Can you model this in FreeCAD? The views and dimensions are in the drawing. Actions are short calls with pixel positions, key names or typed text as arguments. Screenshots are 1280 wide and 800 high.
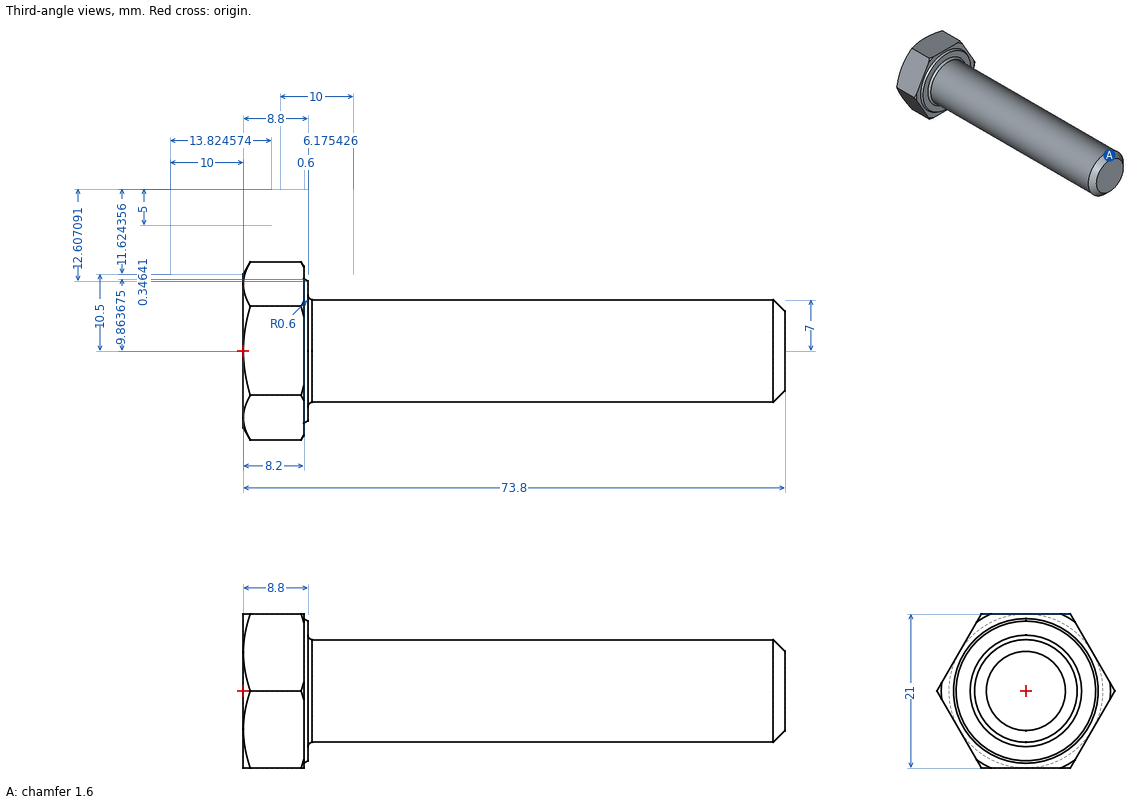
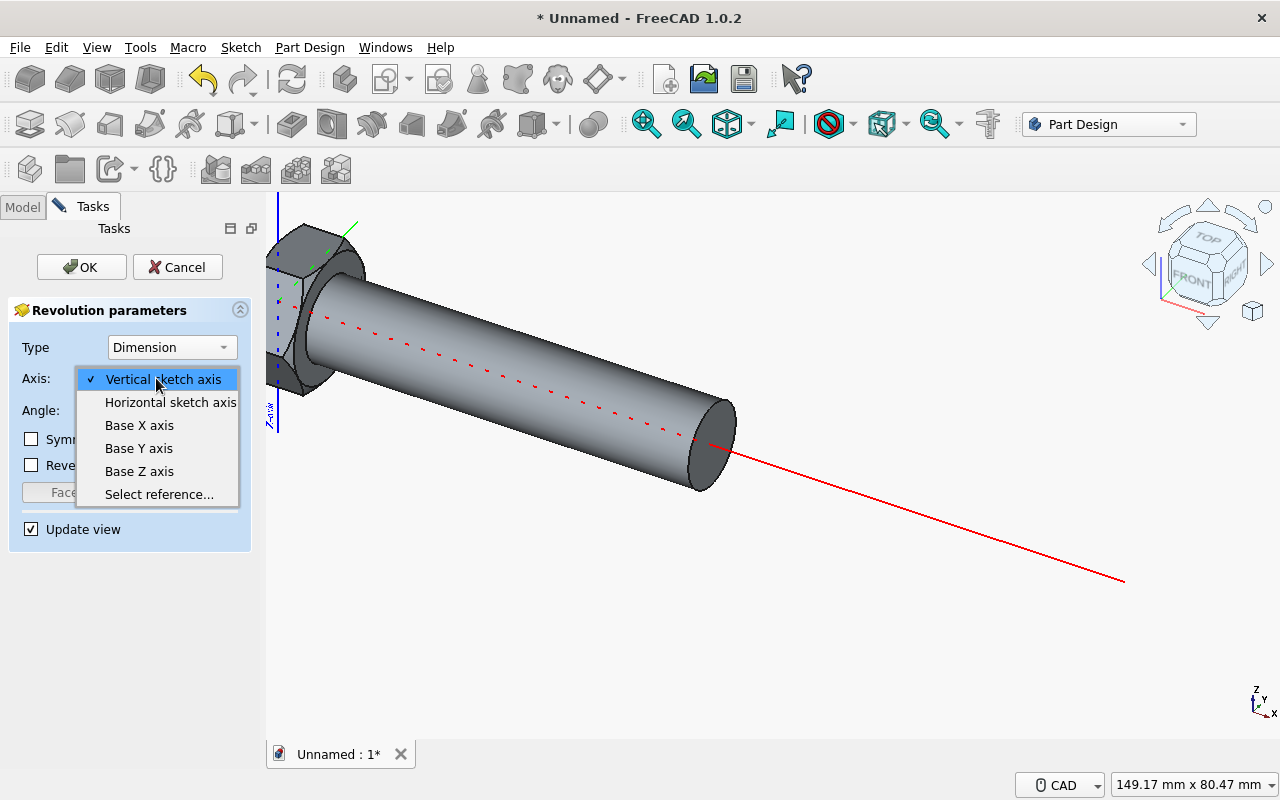
click(156, 402)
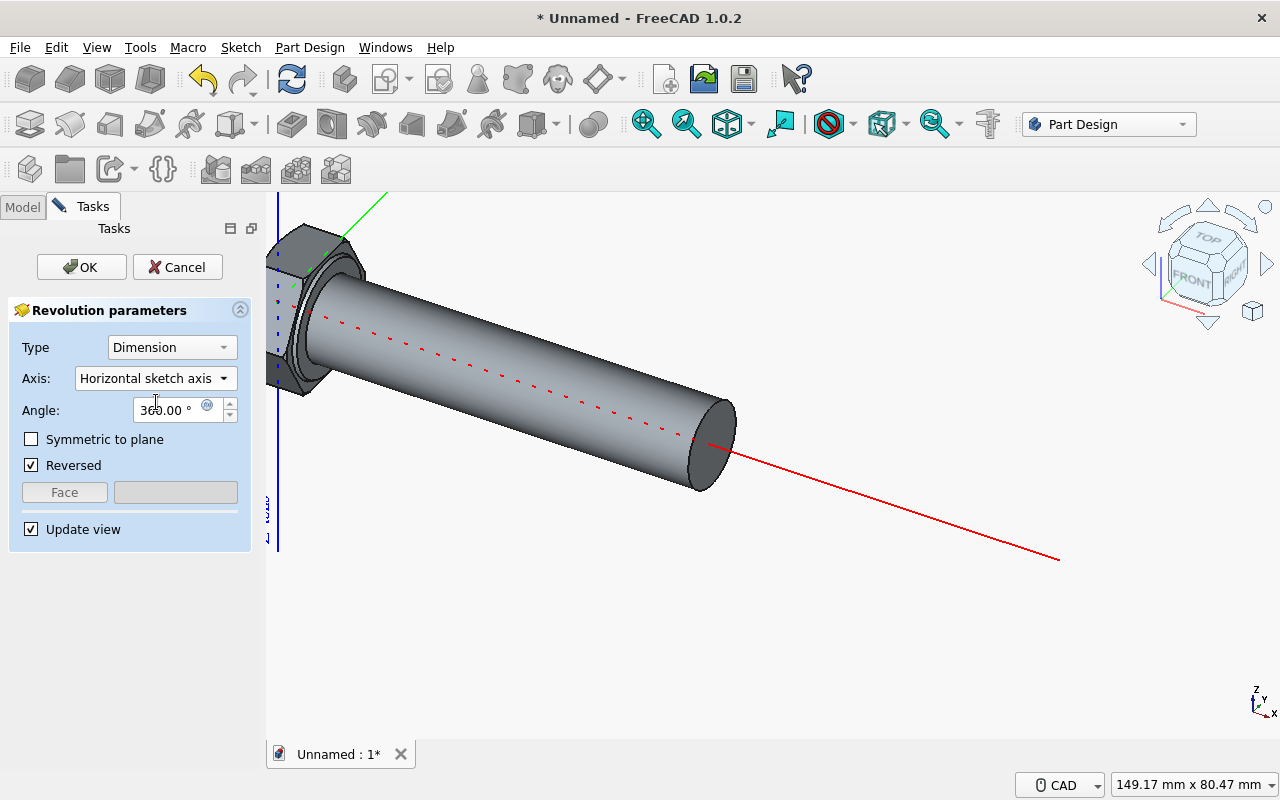
click(82, 267)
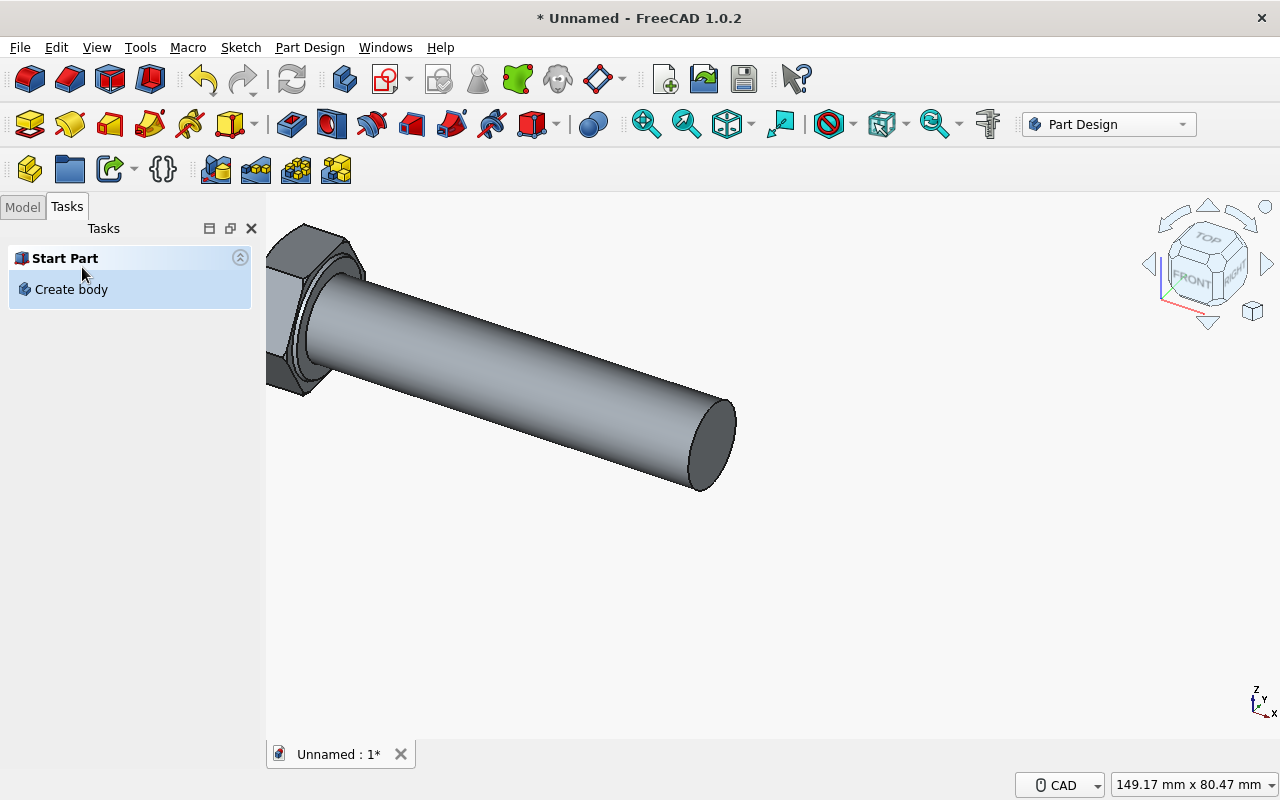
click(648, 124)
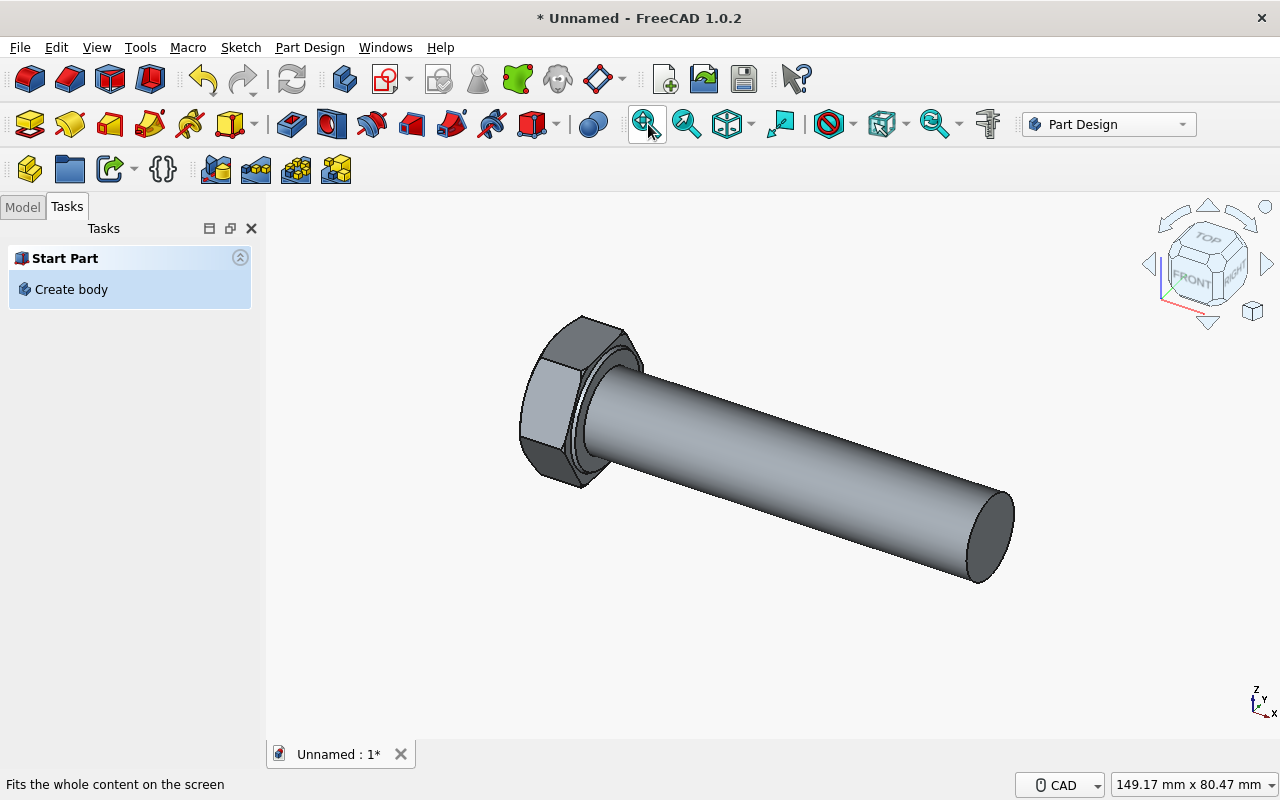
click(966, 560)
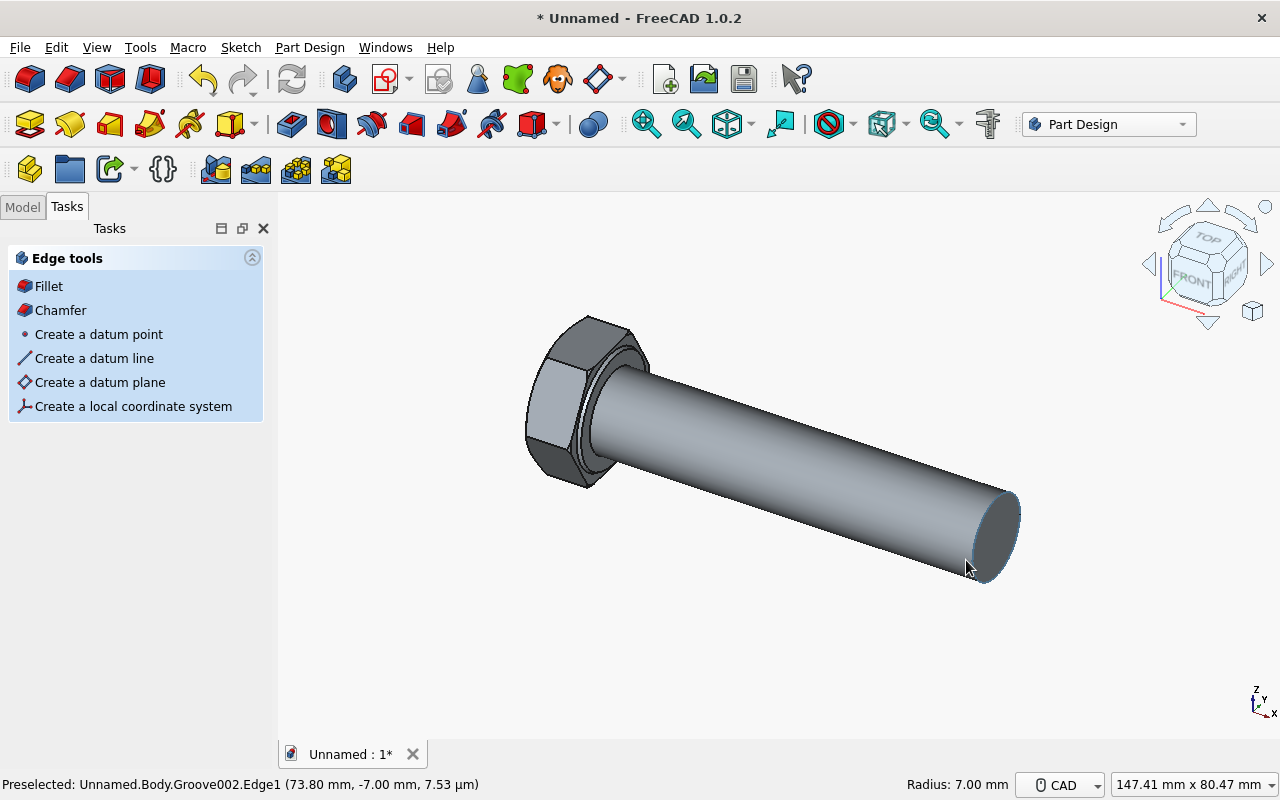
click(70, 80)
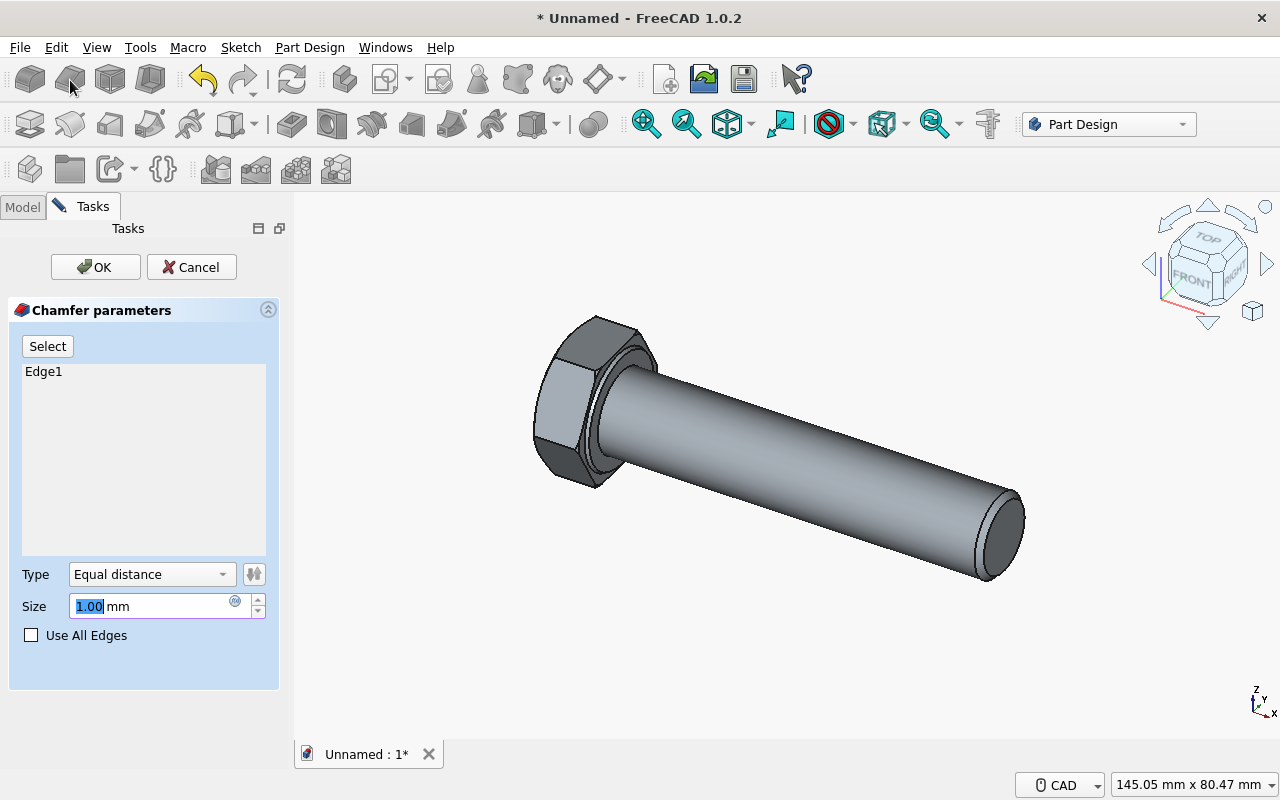
text(1.6)
key(Tab)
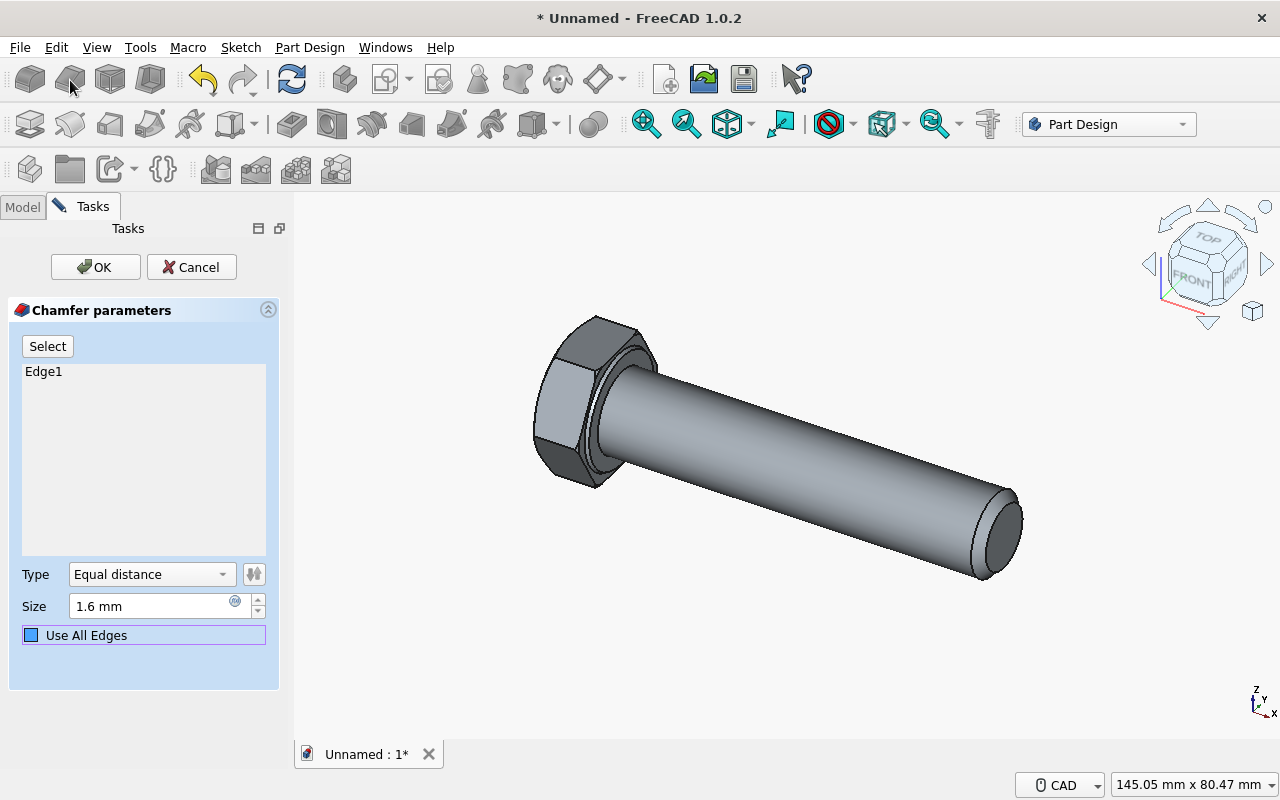
click(96, 267)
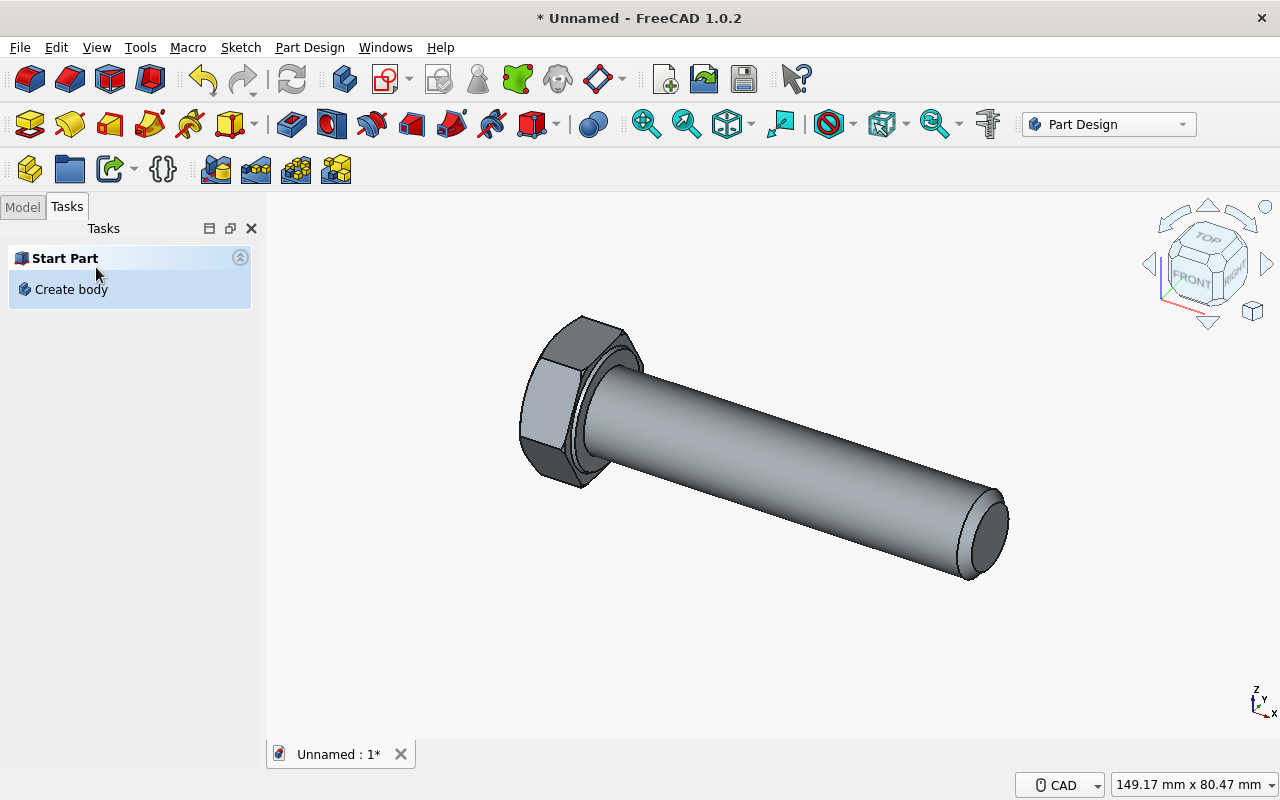
click(386, 80)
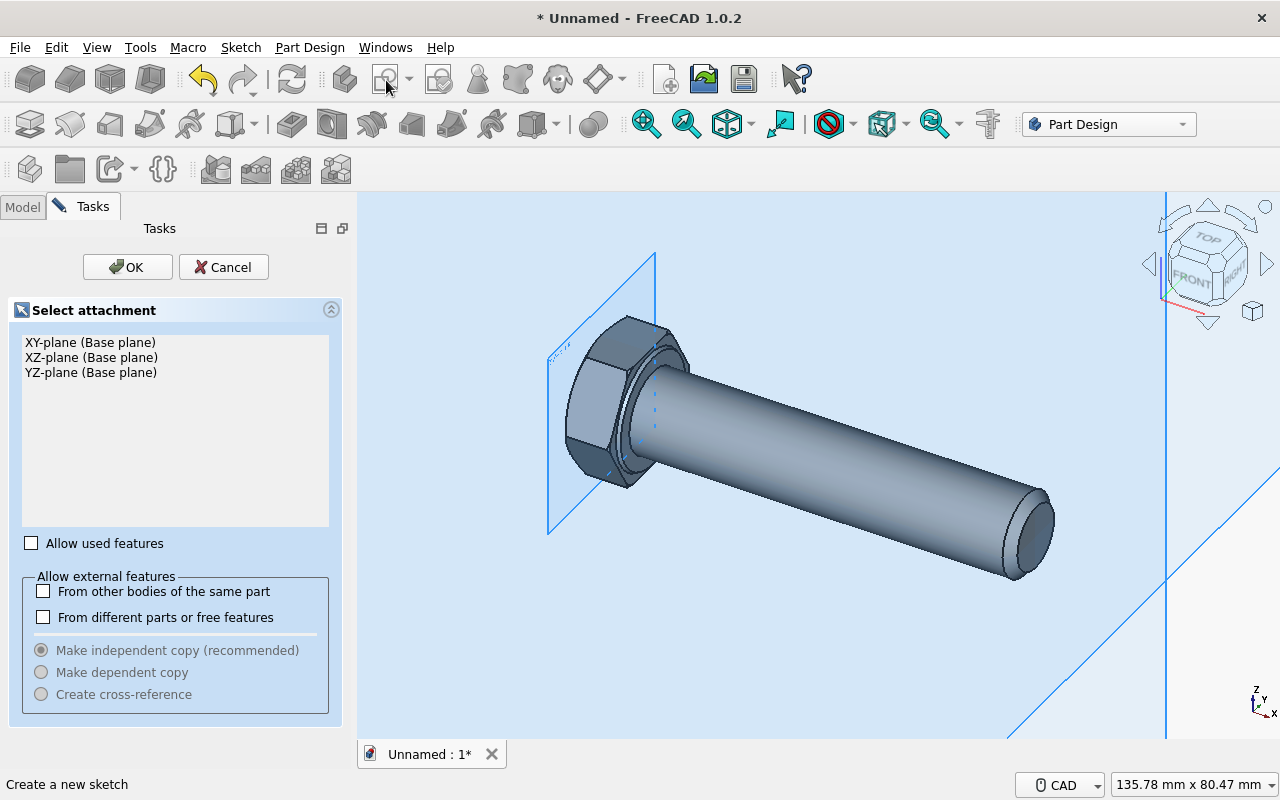
click(82, 342)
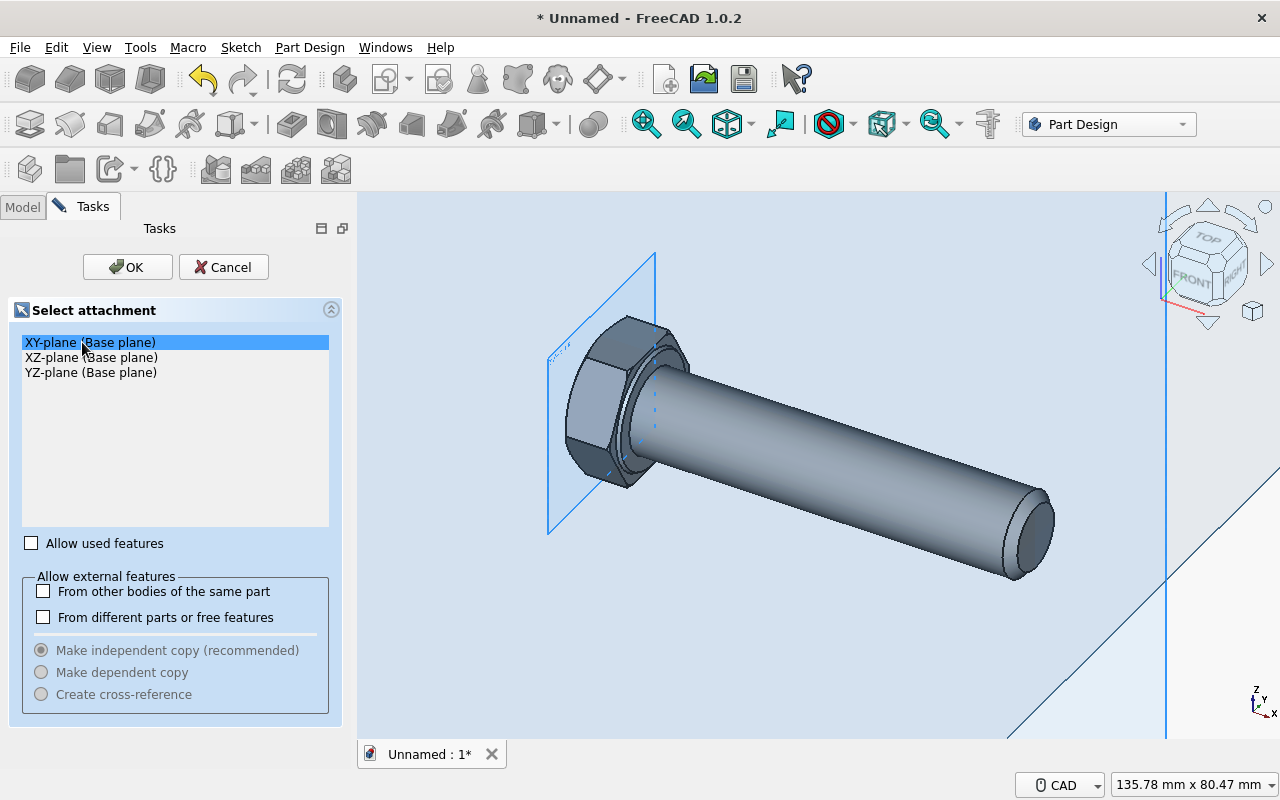
click(128, 267)